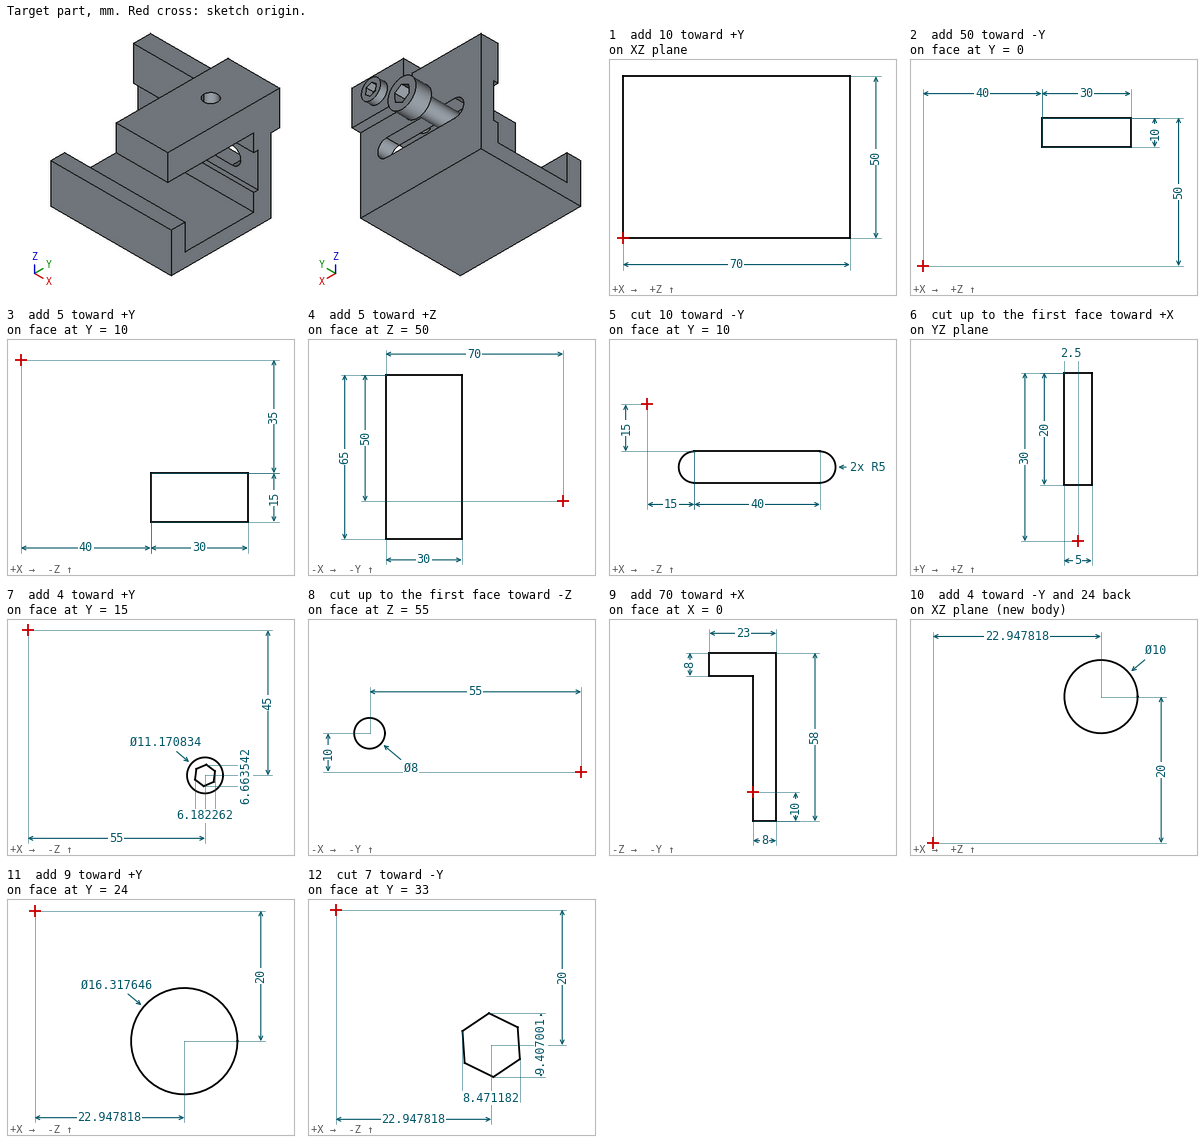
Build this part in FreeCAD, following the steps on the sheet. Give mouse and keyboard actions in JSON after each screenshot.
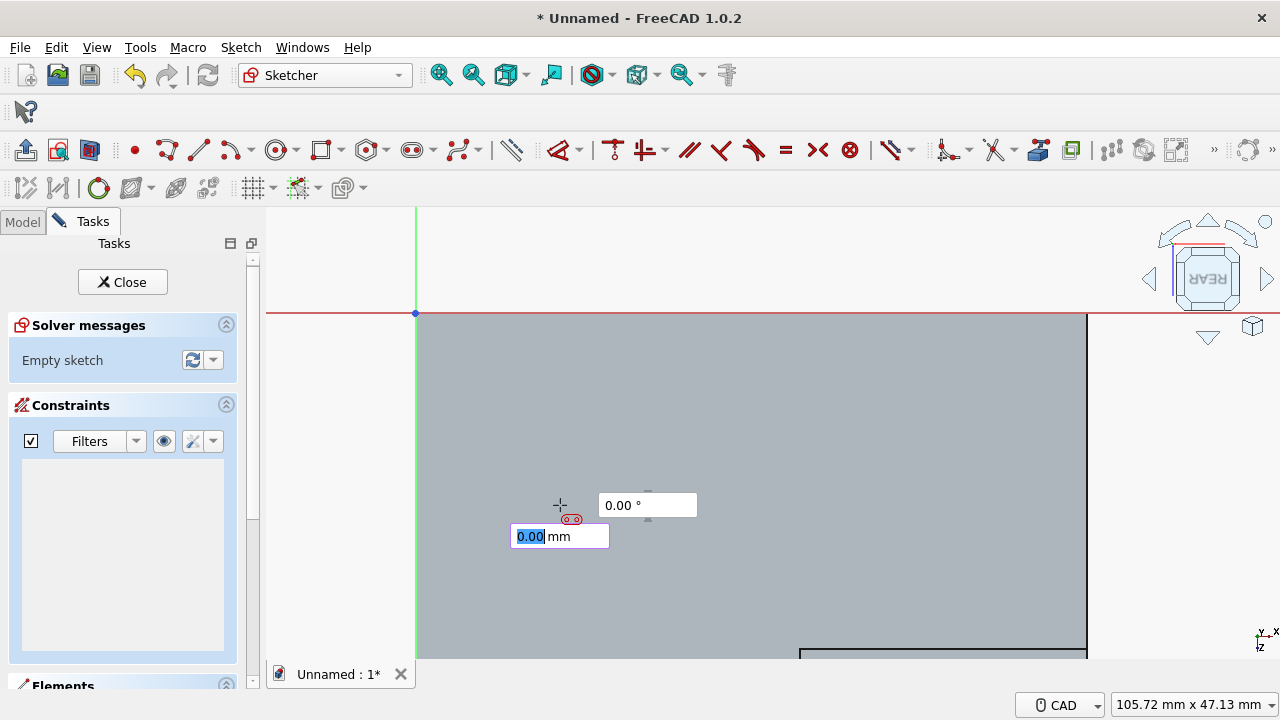
{"action": "left_click", "coordinate": [943, 505]}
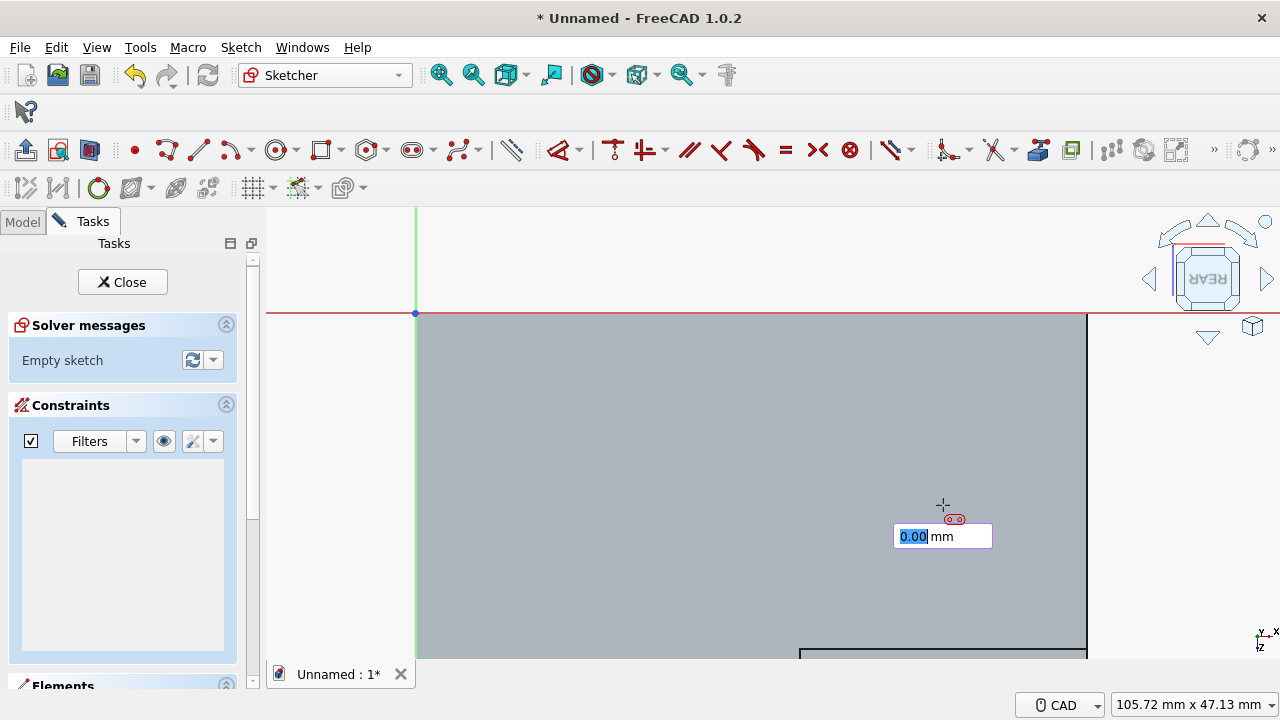
{"action": "left_click", "coordinate": [752, 457]}
{"action": "key", "text": "Escape"}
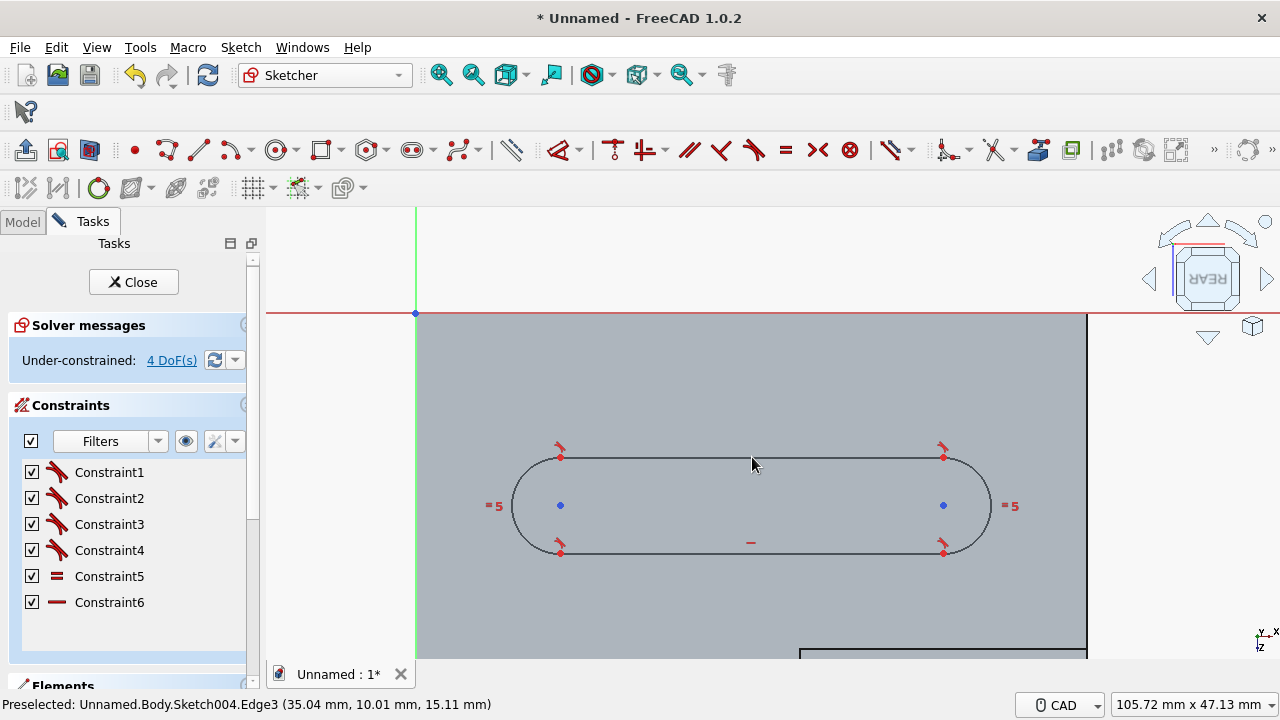
{"action": "left_click", "coordinate": [558, 150]}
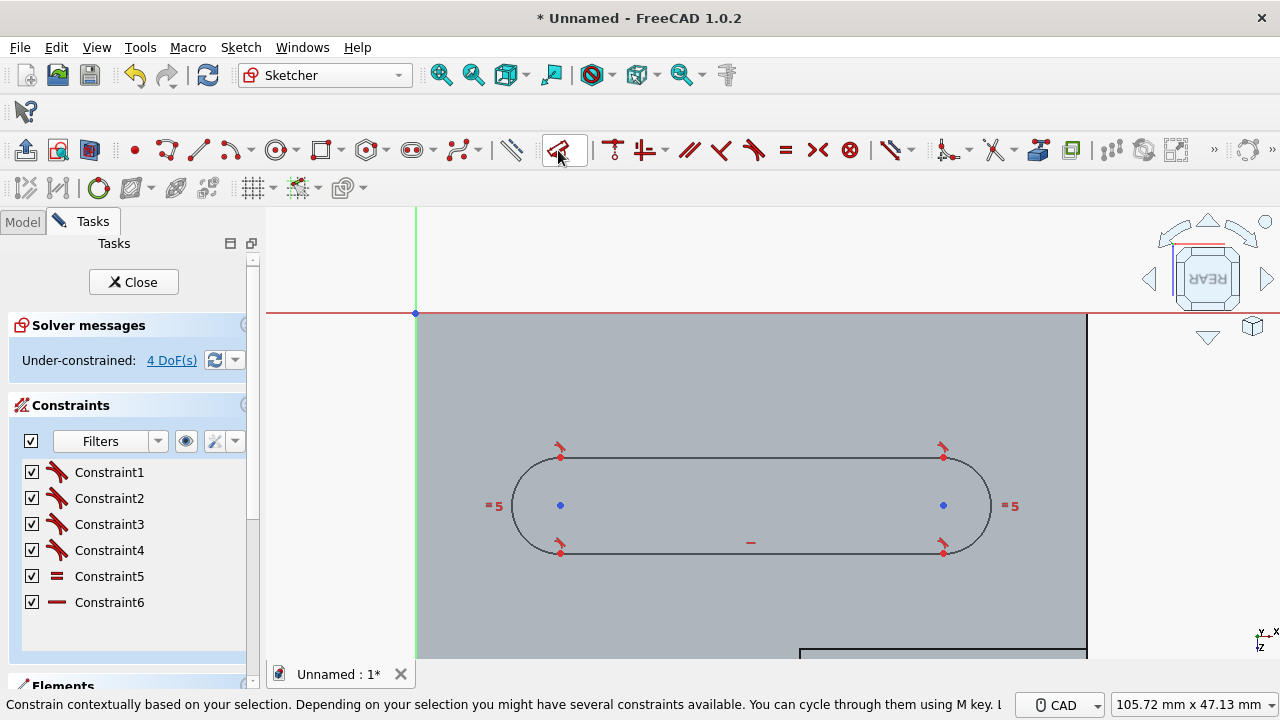
{"action": "left_click", "coordinate": [521, 478]}
{"action": "left_click", "coordinate": [495, 459]}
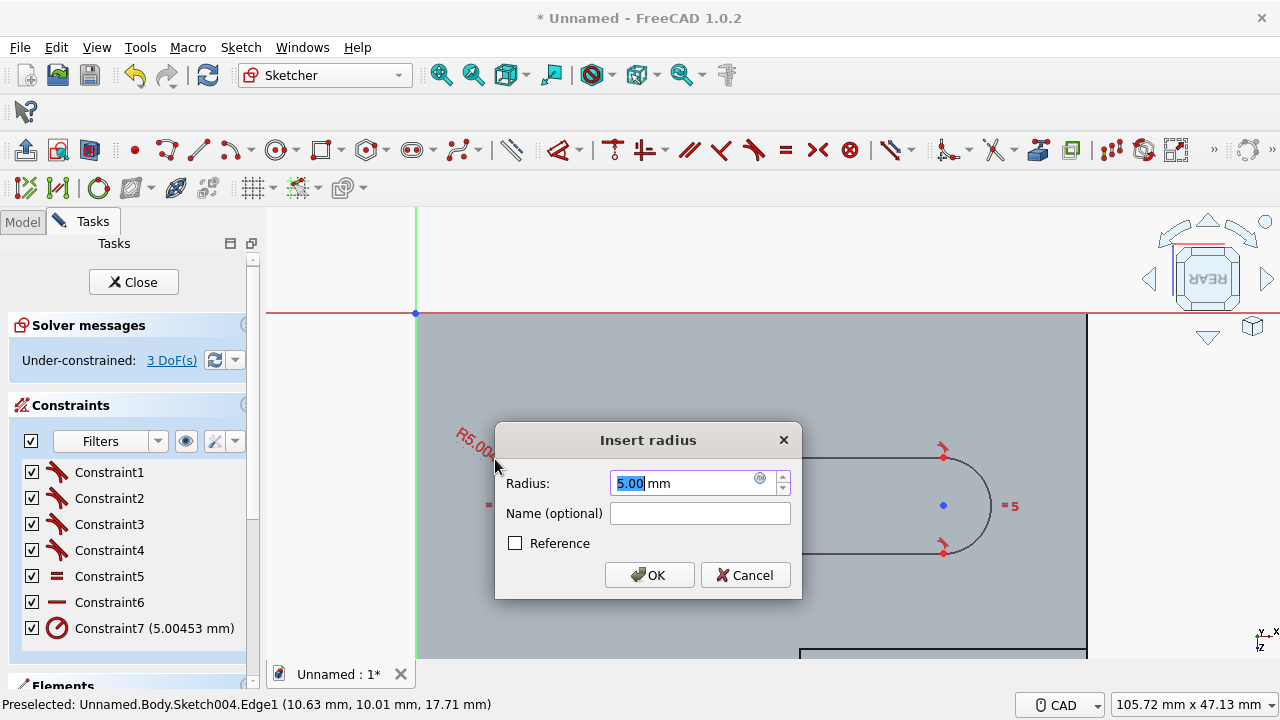
{"action": "type", "text": "5"}
{"action": "key", "text": "Return"}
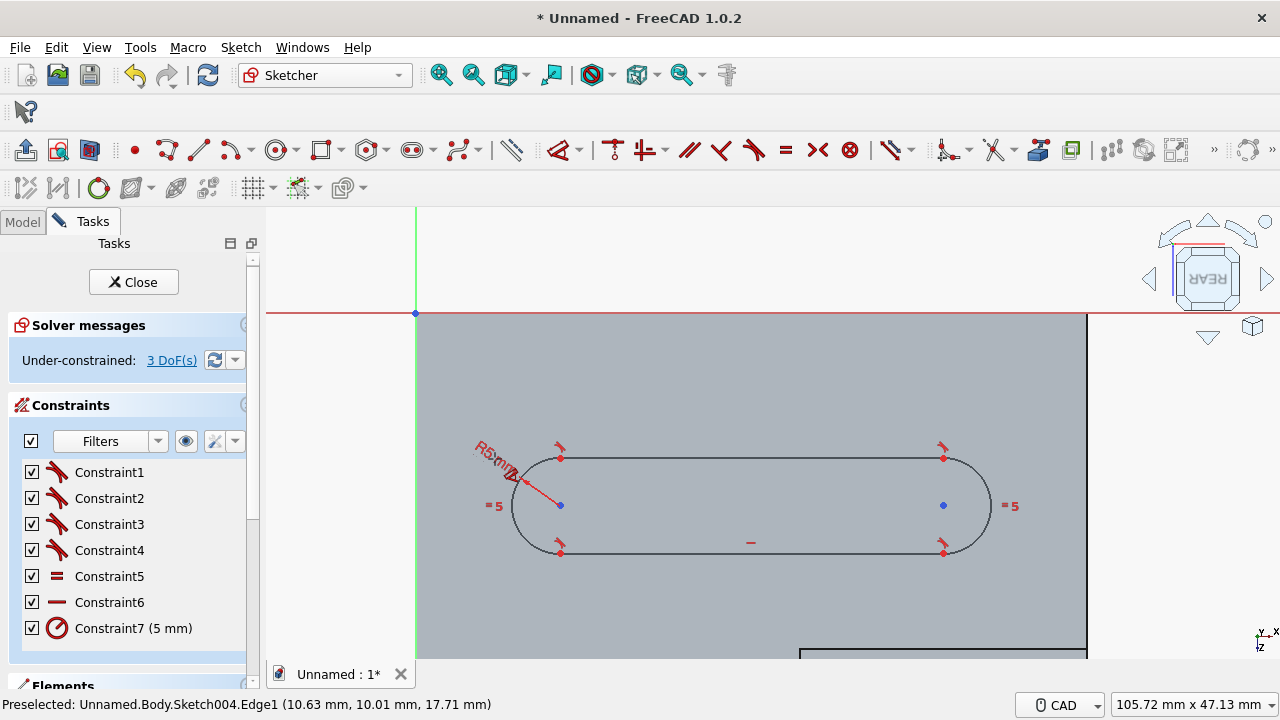
{"action": "left_click", "coordinate": [675, 458]}
{"action": "left_click", "coordinate": [752, 492]}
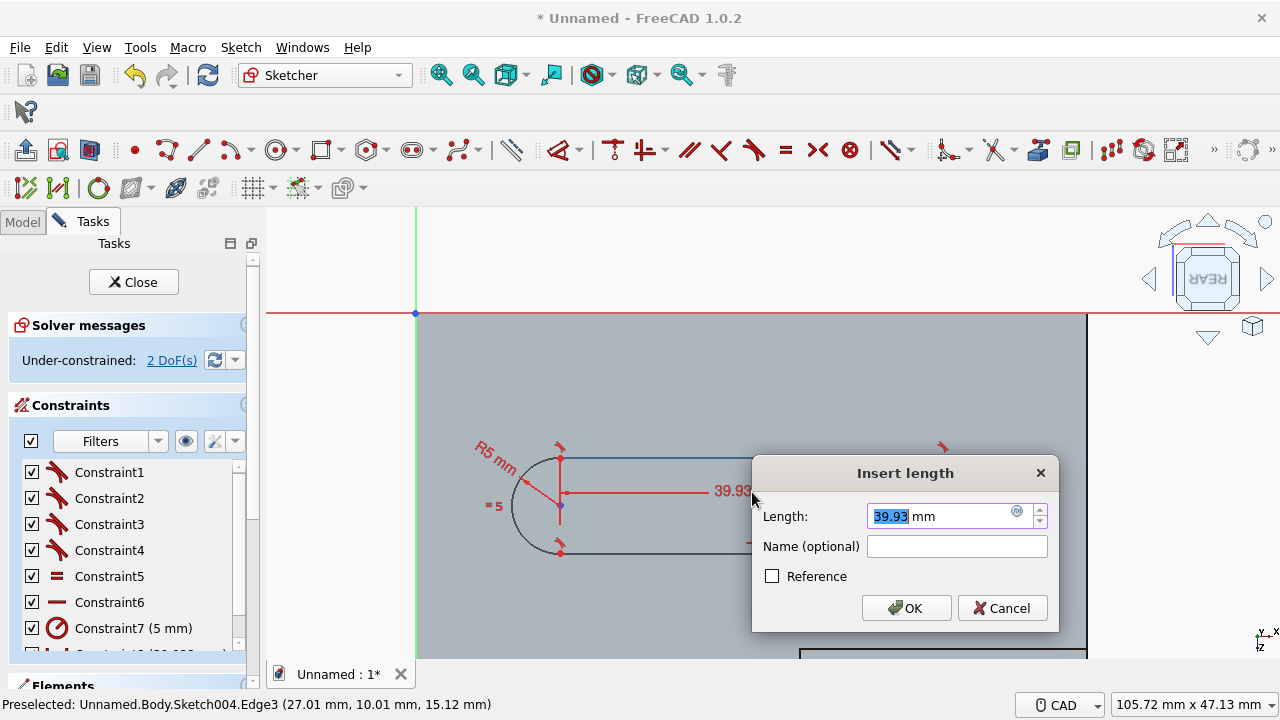
{"action": "type", "text": "40"}
{"action": "key", "text": "Return"}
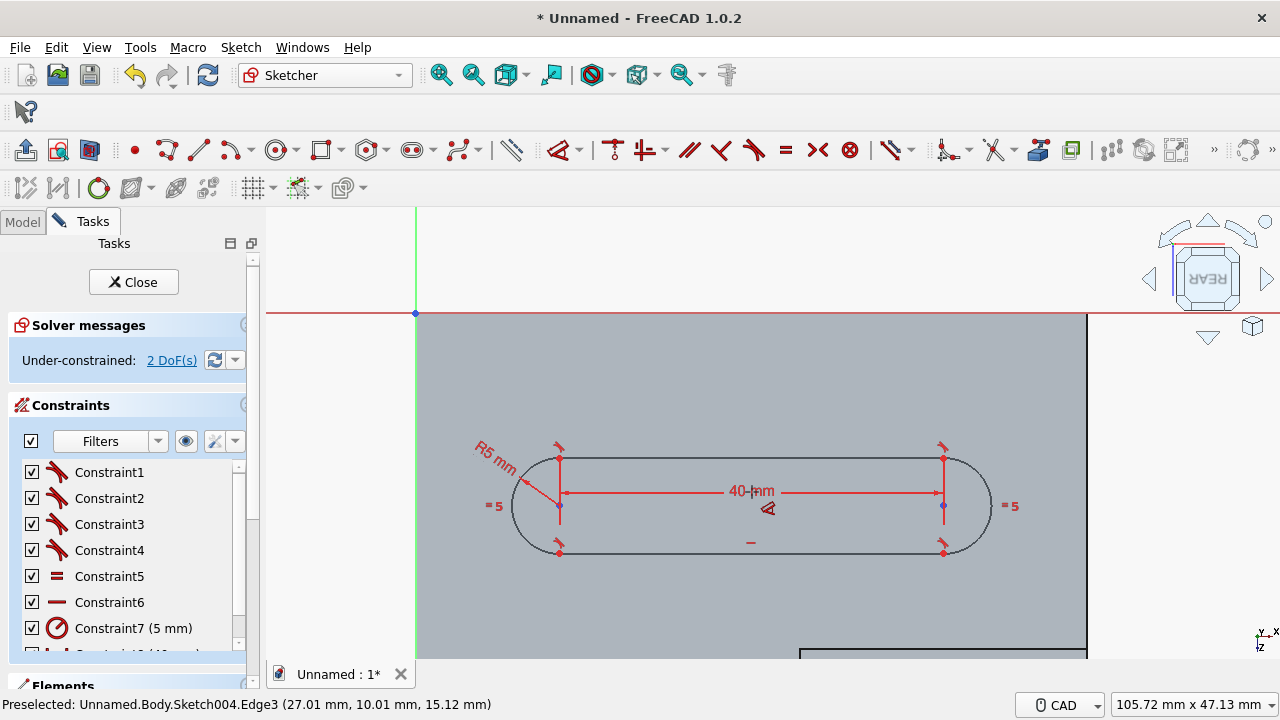
{"action": "left_click", "coordinate": [560, 458]}
{"action": "left_click", "coordinate": [488, 279]}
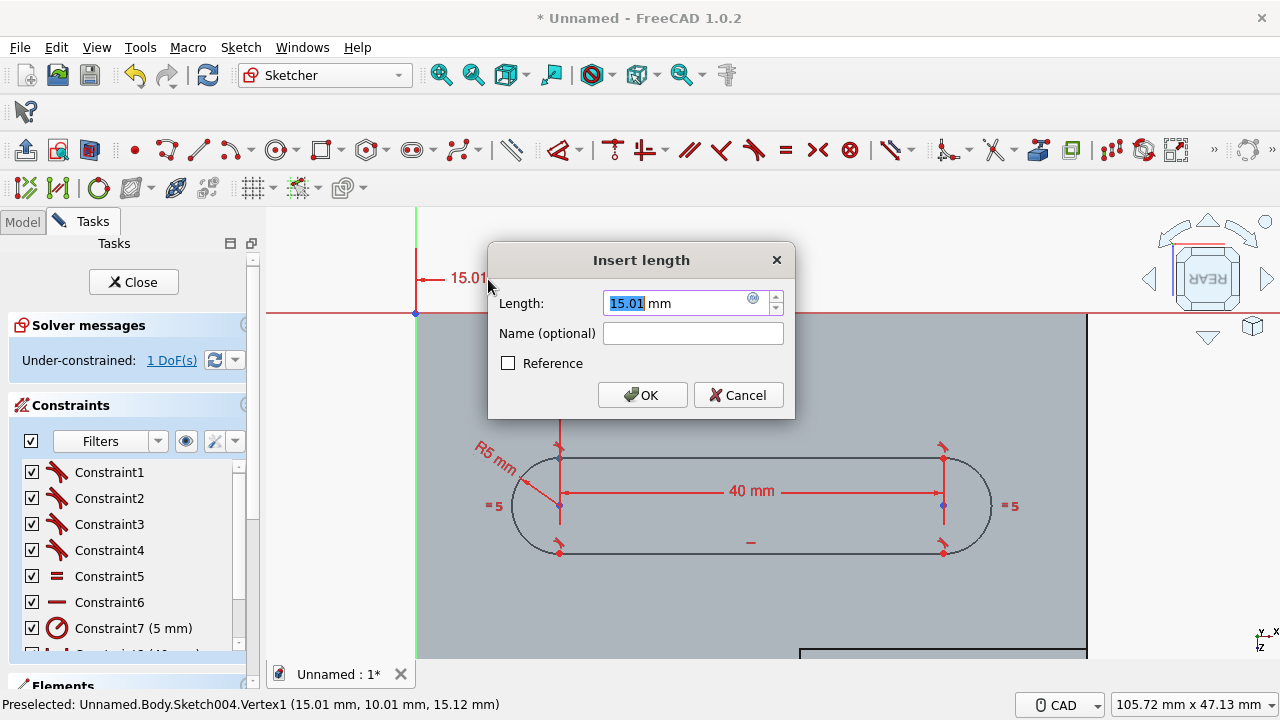
{"action": "type", "text": "15"}
{"action": "key", "text": "Return"}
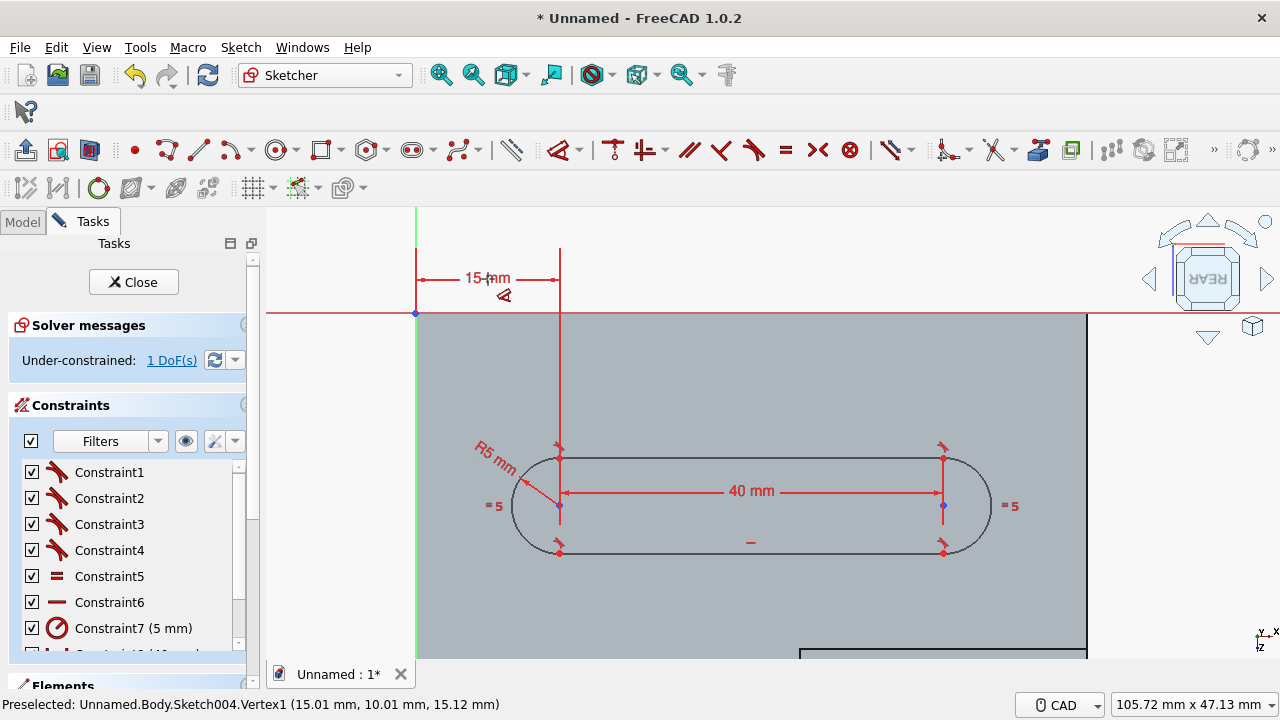
{"action": "left_click", "coordinate": [560, 458]}
{"action": "left_click", "coordinate": [382, 386]}